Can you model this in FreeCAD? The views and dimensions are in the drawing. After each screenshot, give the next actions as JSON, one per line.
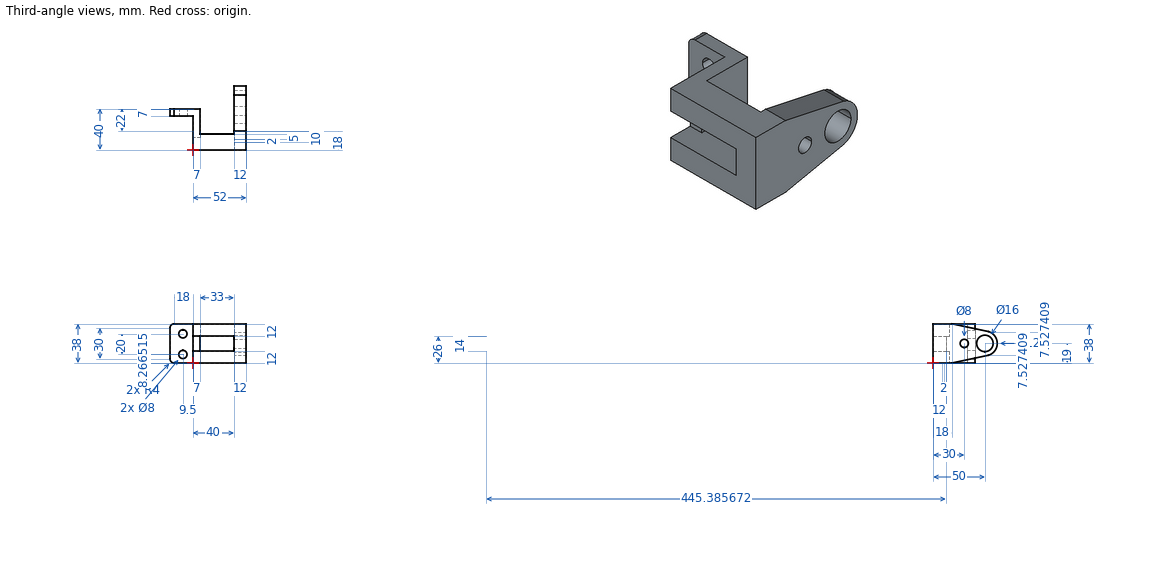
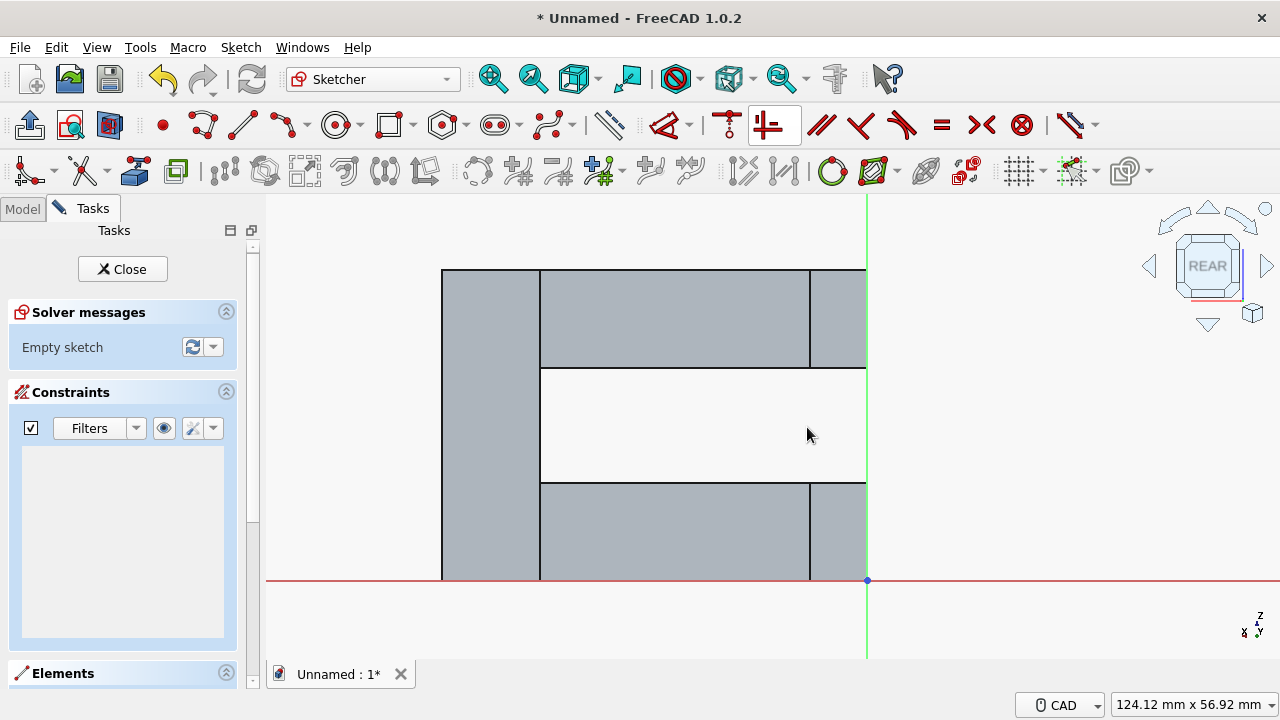
{"action": "left_click", "coordinate": [390, 126]}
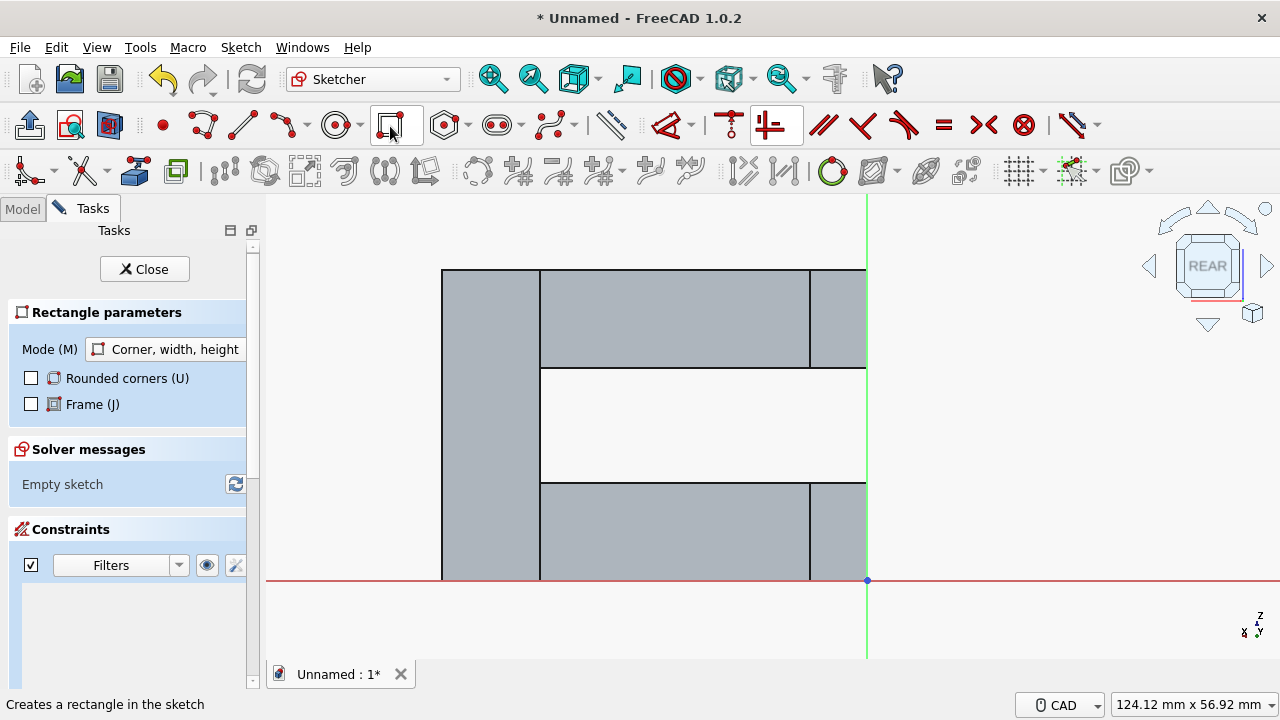
{"action": "left_click", "coordinate": [540, 270]}
{"action": "left_click", "coordinate": [810, 368]}
{"action": "key", "text": "Escape"}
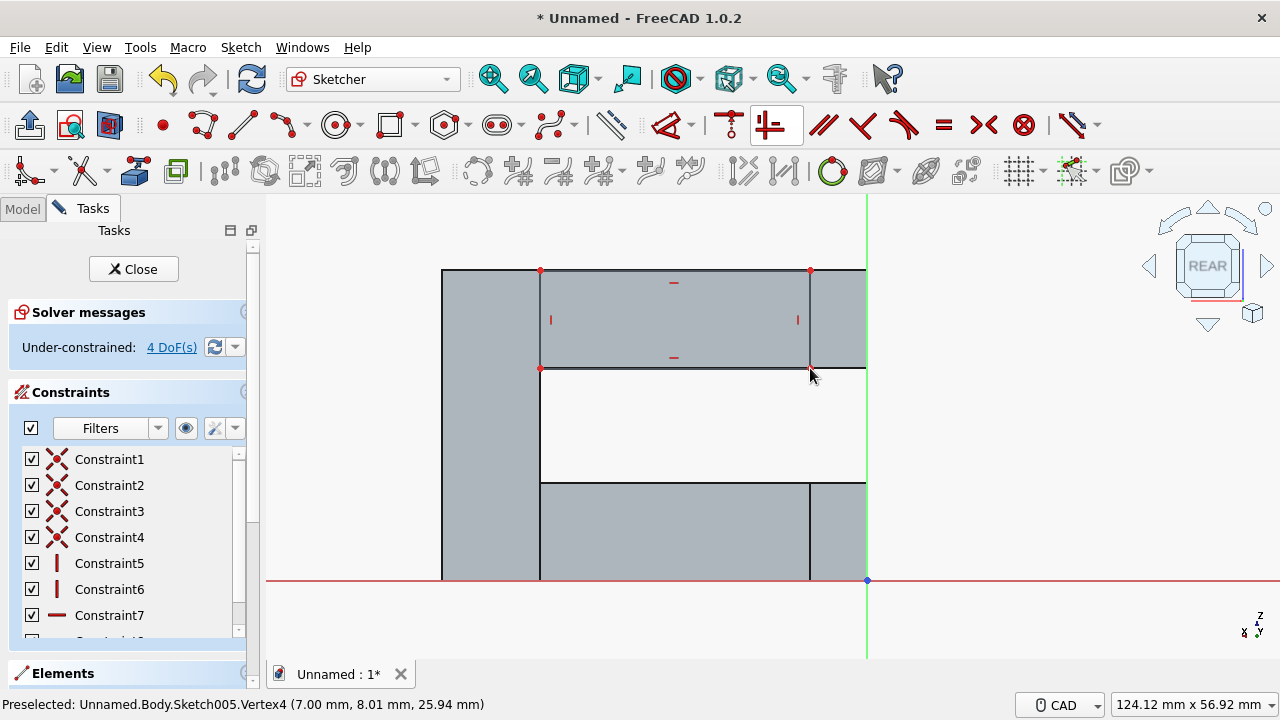
{"action": "left_click", "coordinate": [666, 126]}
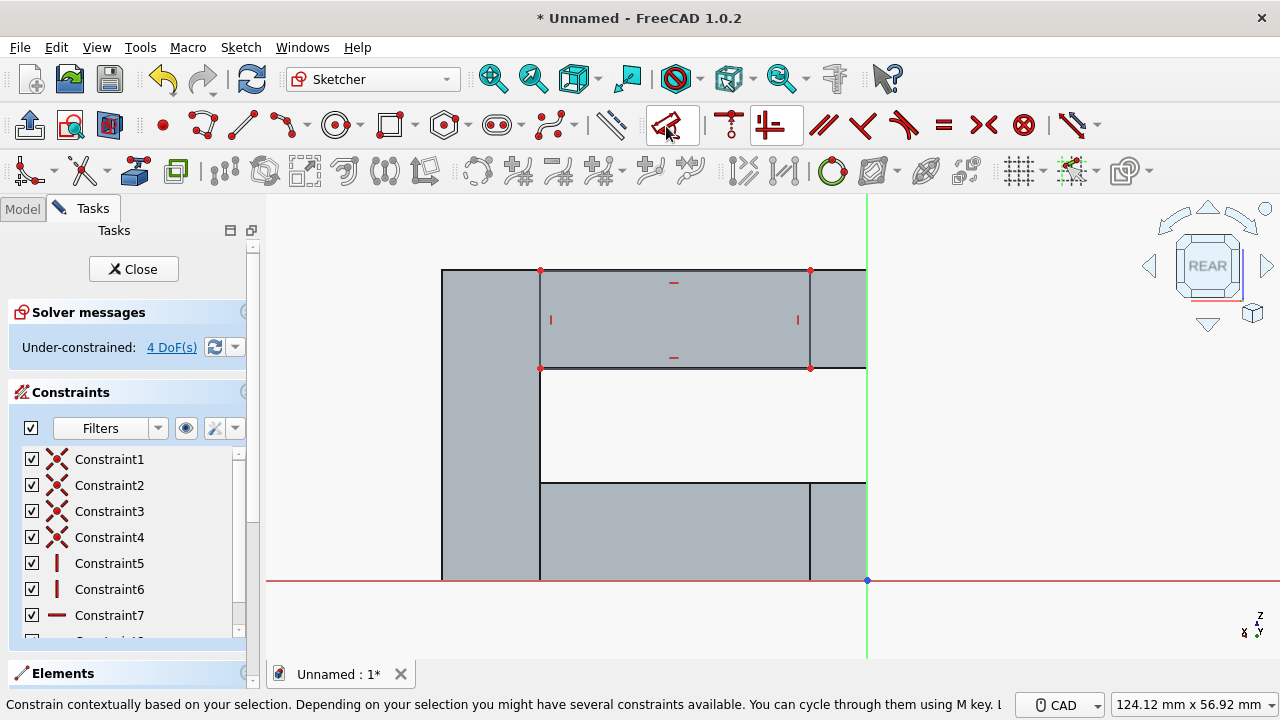
{"action": "left_click", "coordinate": [540, 300]}
{"action": "left_click", "coordinate": [506, 320]}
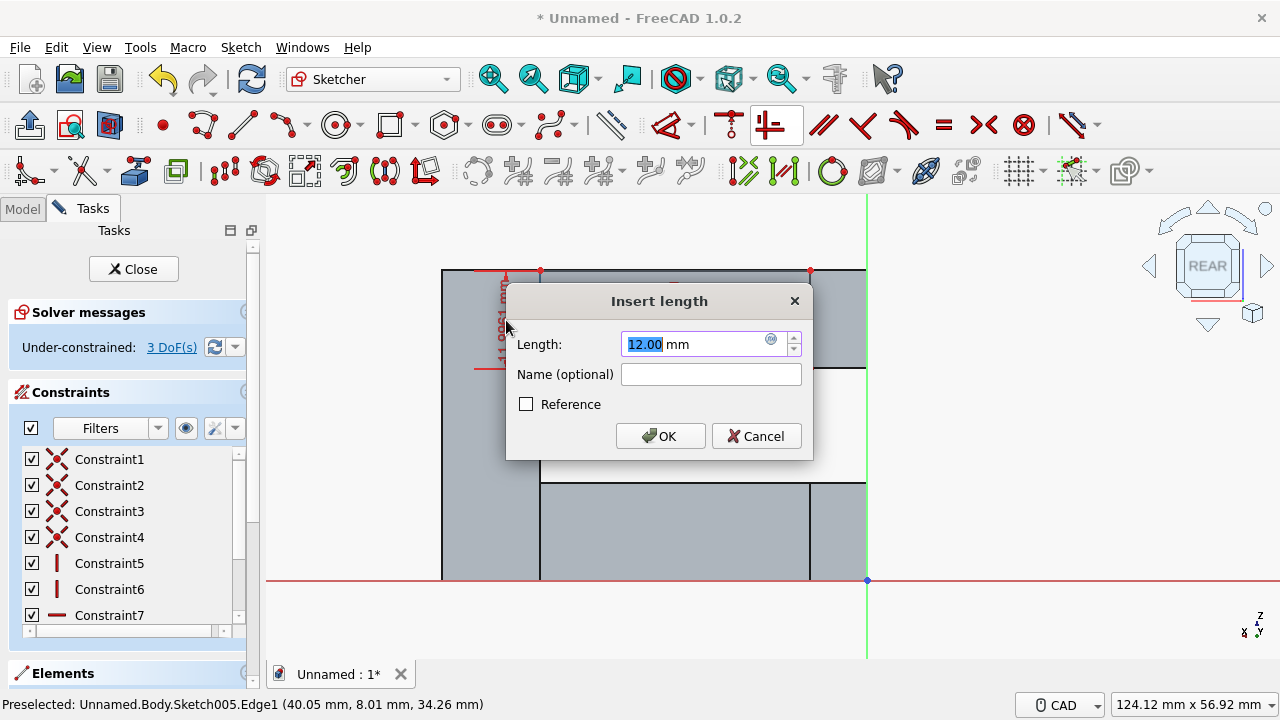
{"action": "type", "text": "12"}
{"action": "key", "text": "Return"}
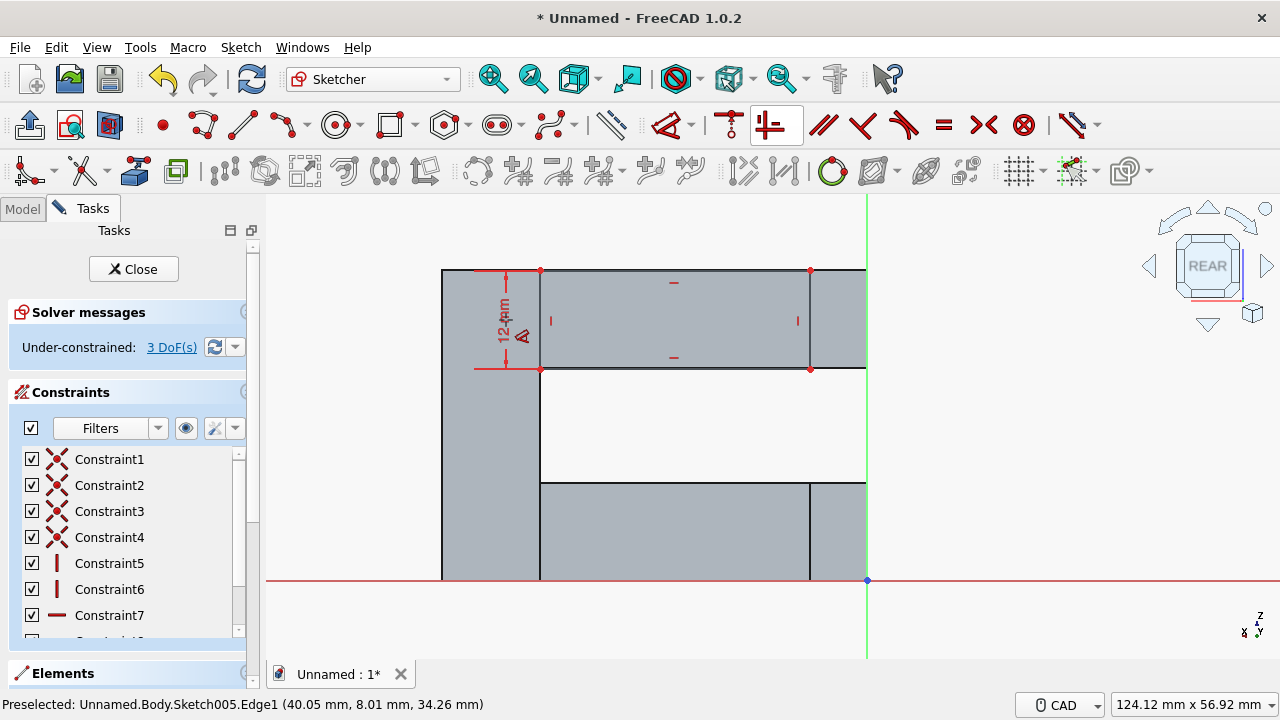
{"action": "left_click", "coordinate": [621, 369]}
{"action": "left_click", "coordinate": [675, 335]}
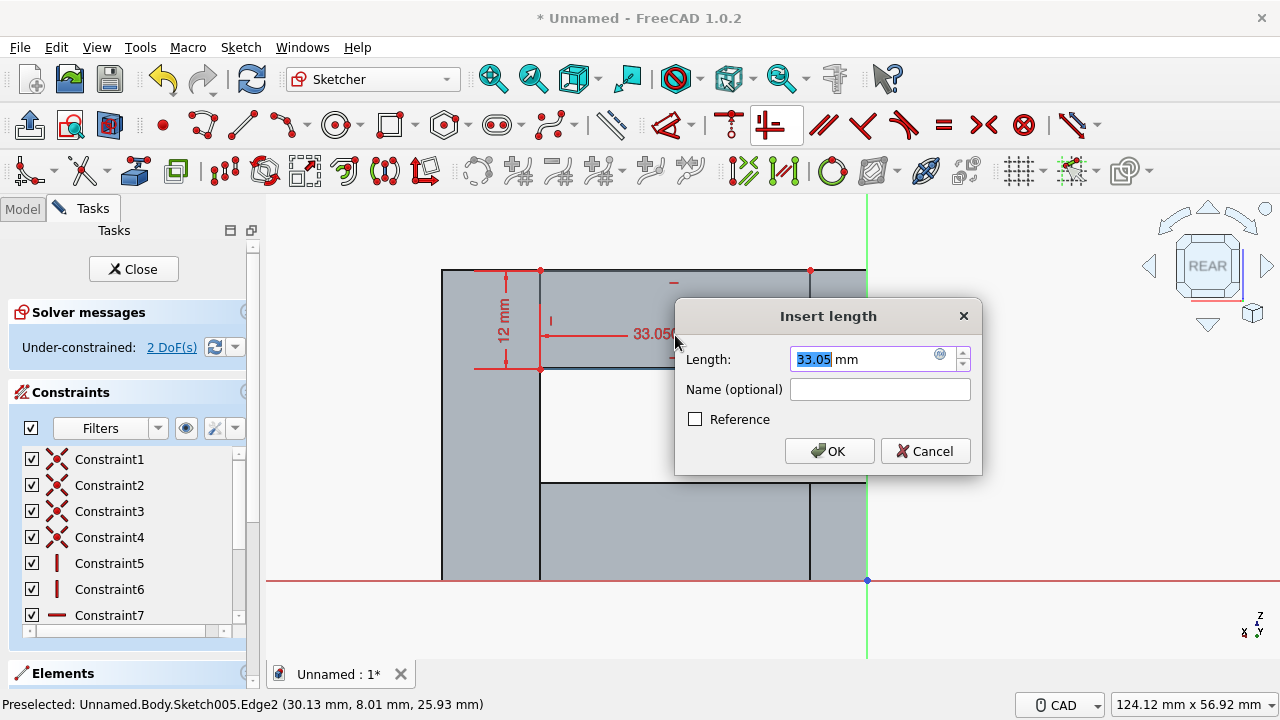
{"action": "type", "text": "33"}
{"action": "key", "text": "Return"}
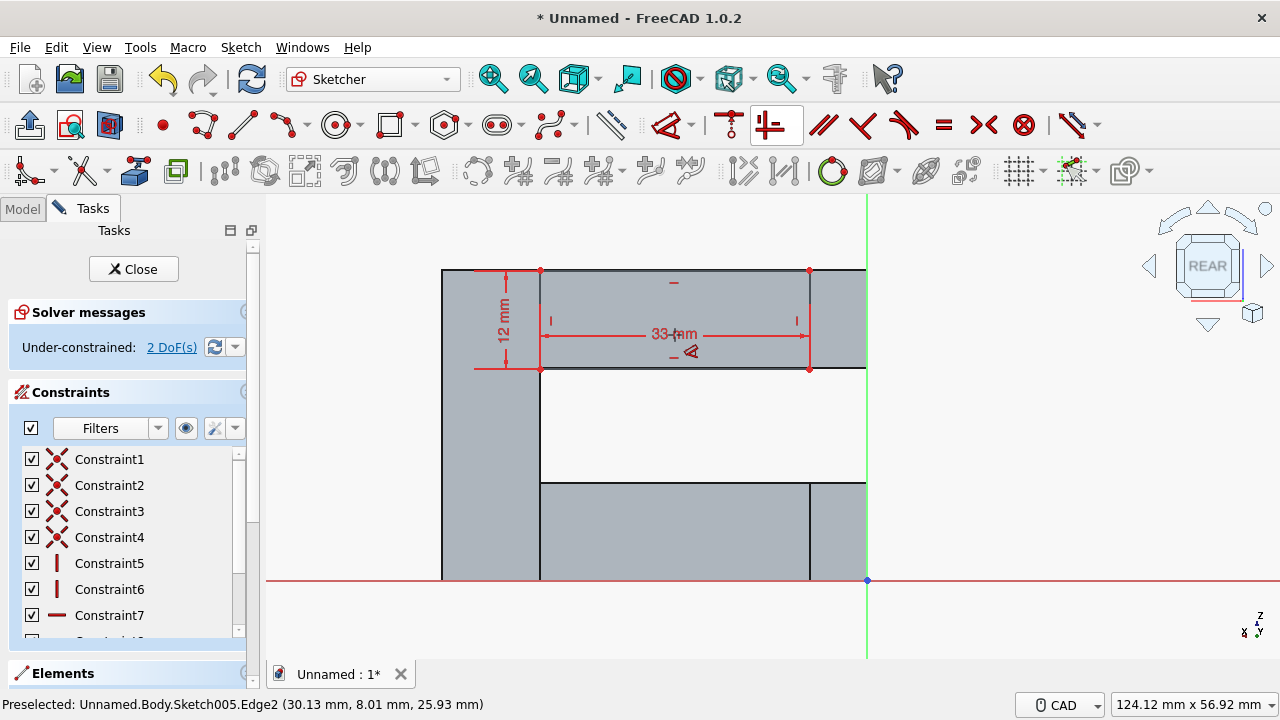
{"action": "left_click", "coordinate": [810, 369]}
{"action": "left_click", "coordinate": [838, 615]}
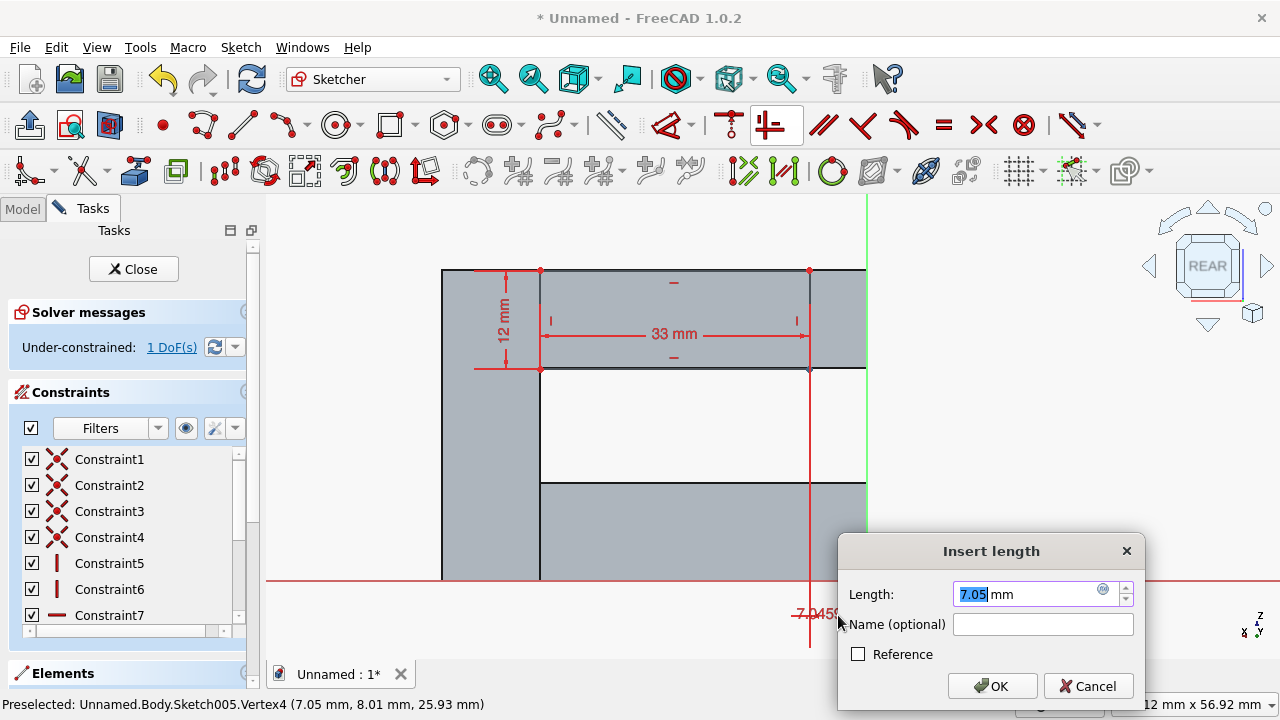
{"action": "type", "text": "7"}
{"action": "key", "text": "Return"}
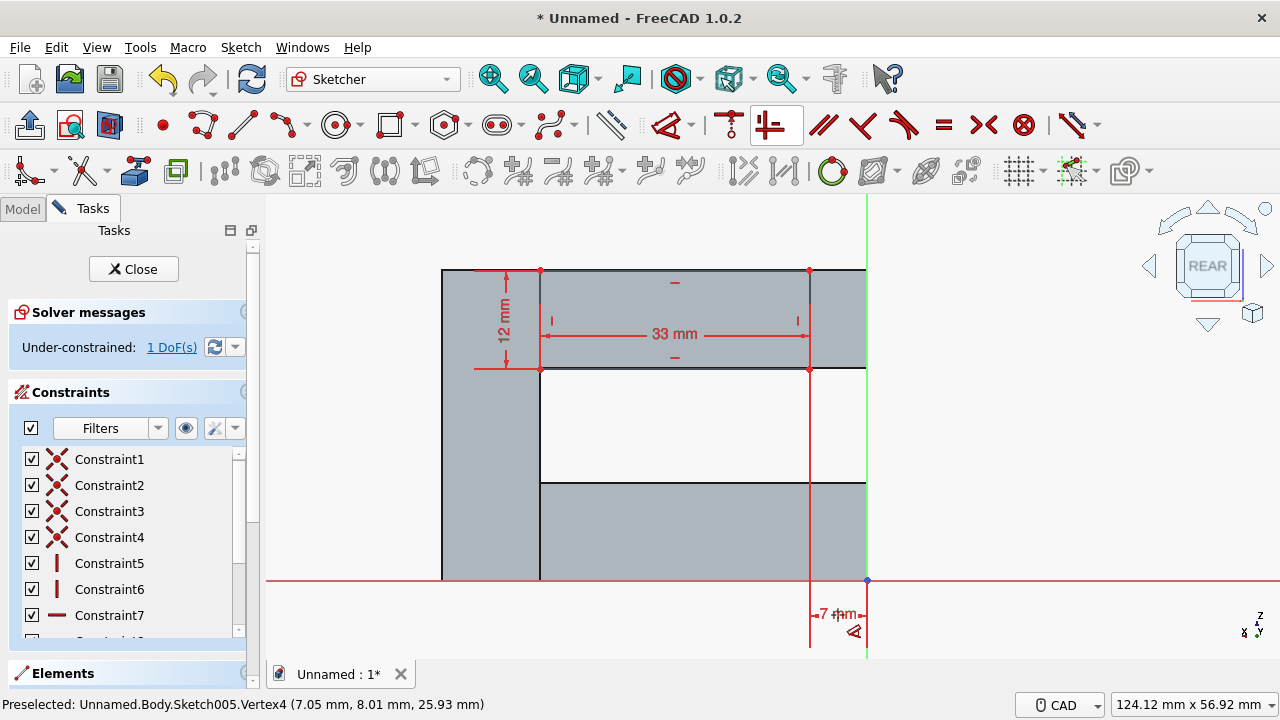
{"action": "left_click", "coordinate": [540, 271]}
{"action": "left_click", "coordinate": [506, 426]}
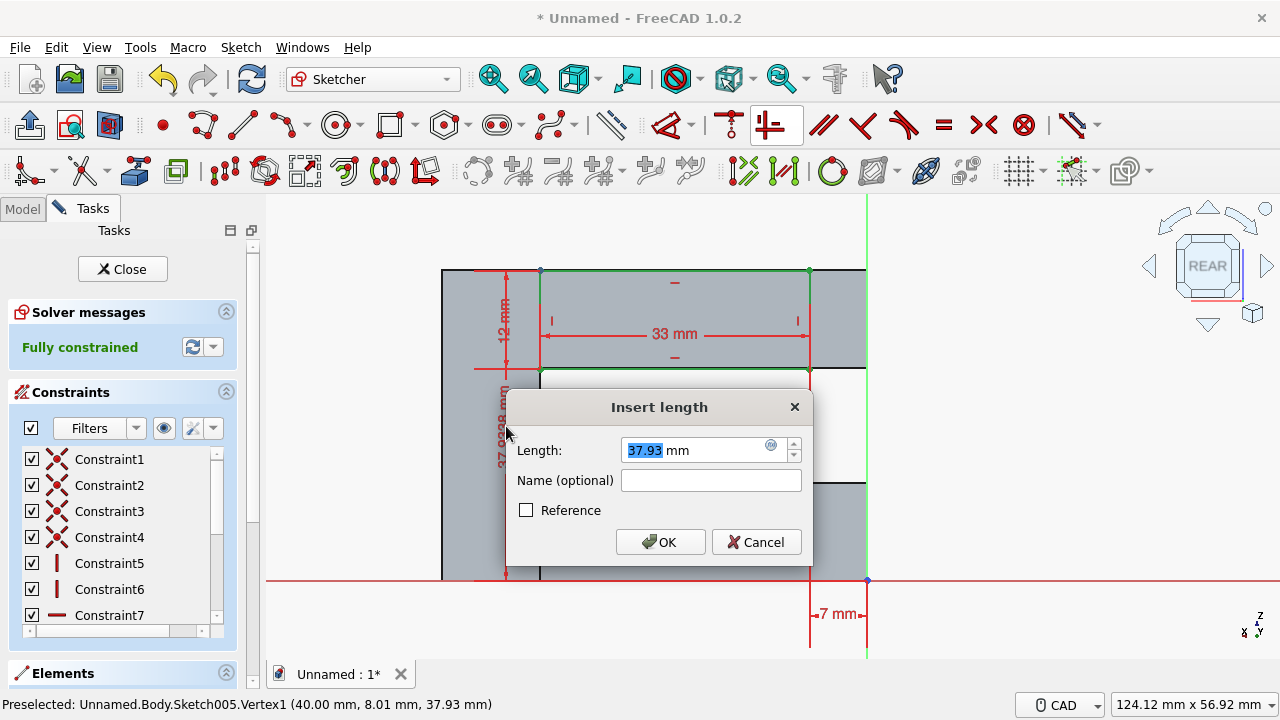
{"action": "type", "text": "38"}
{"action": "key", "text": "Return"}
{"action": "key", "text": "Escape"}